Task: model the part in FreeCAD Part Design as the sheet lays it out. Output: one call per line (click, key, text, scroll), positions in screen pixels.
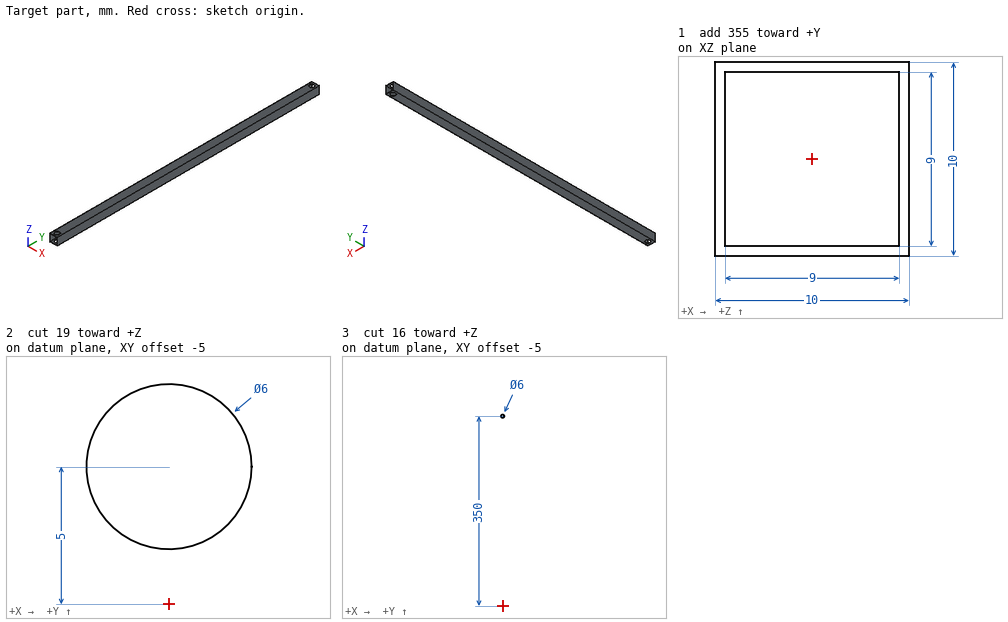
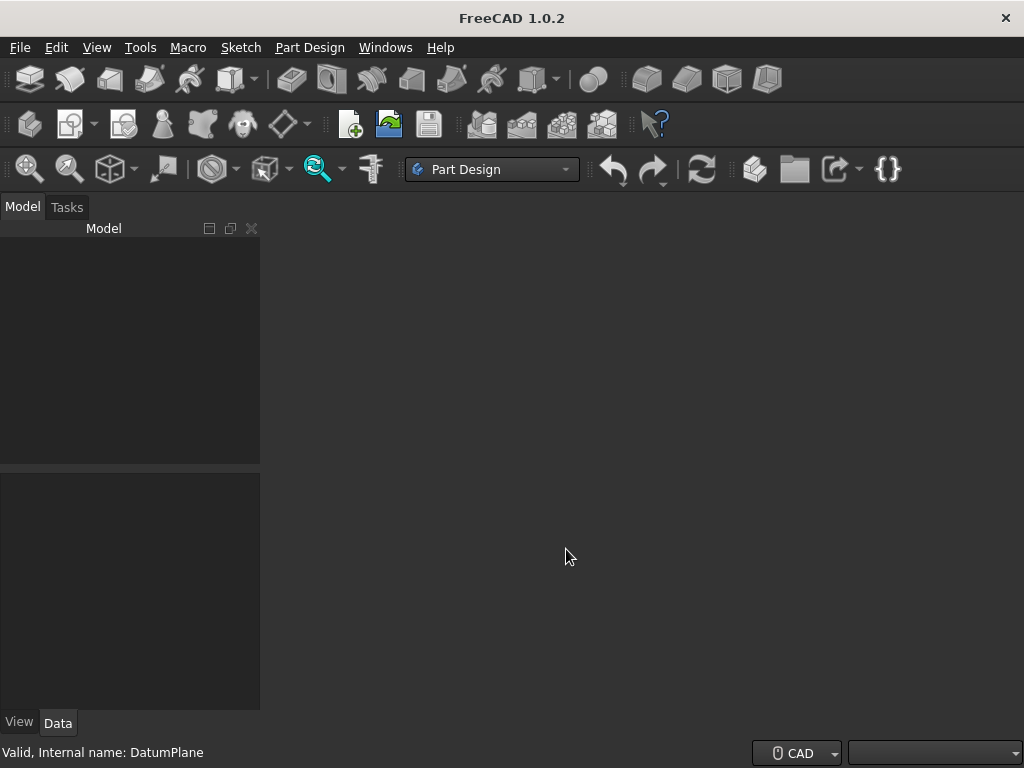
key(ctrl+n)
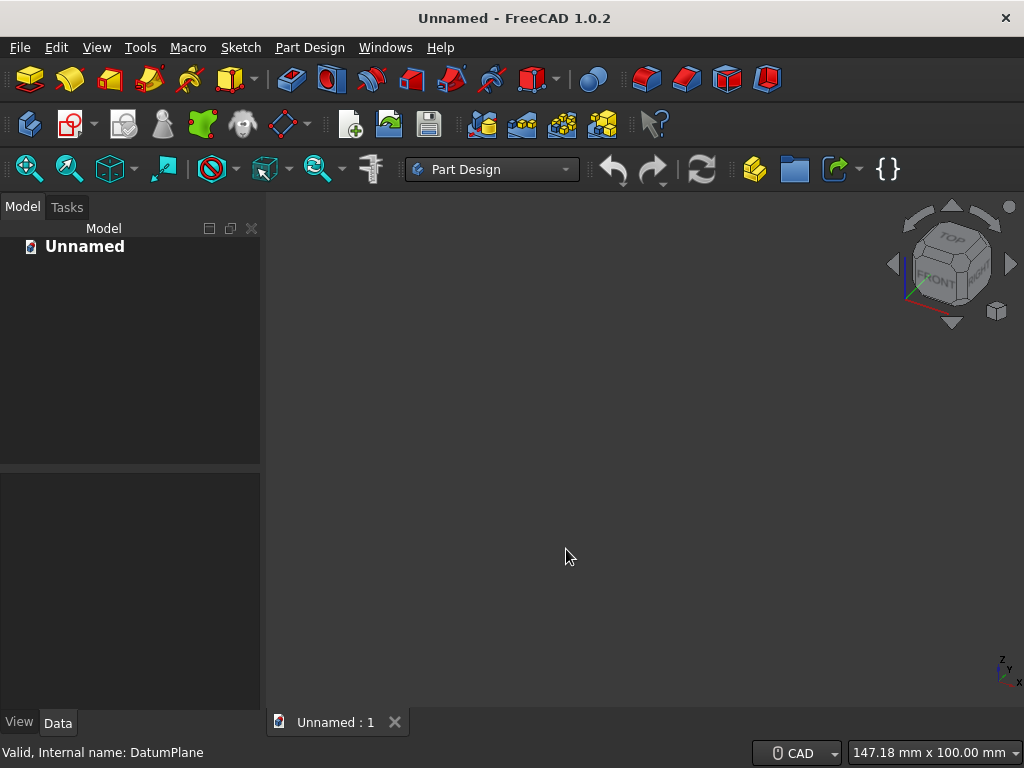
click(70, 124)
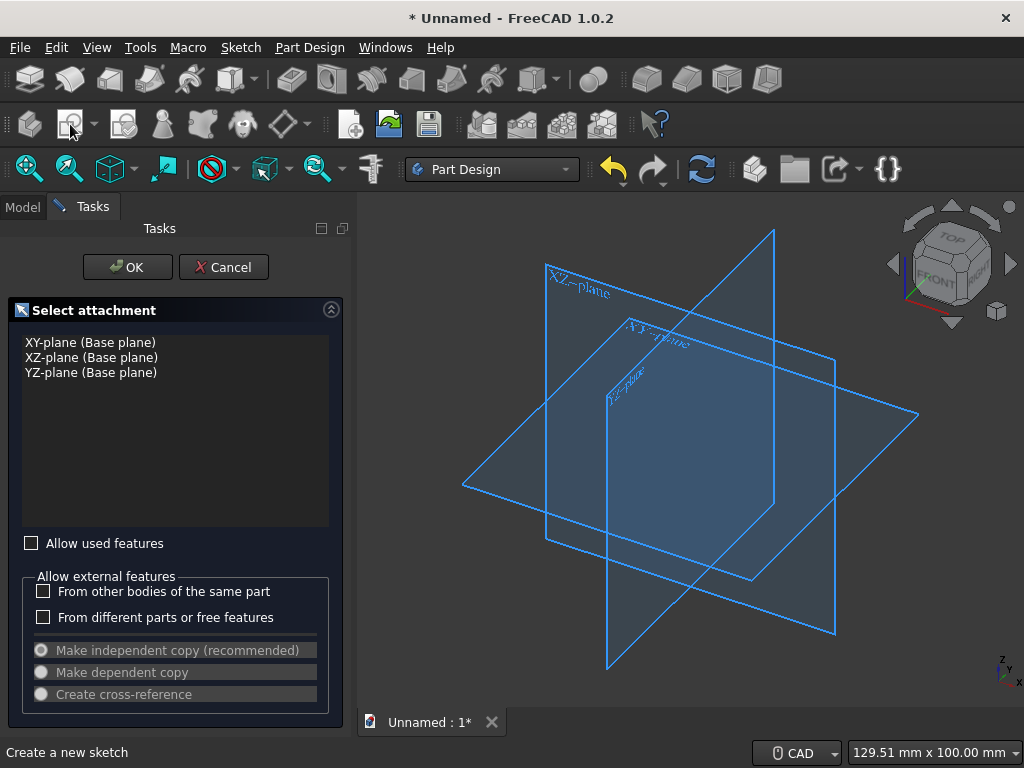
click(82, 358)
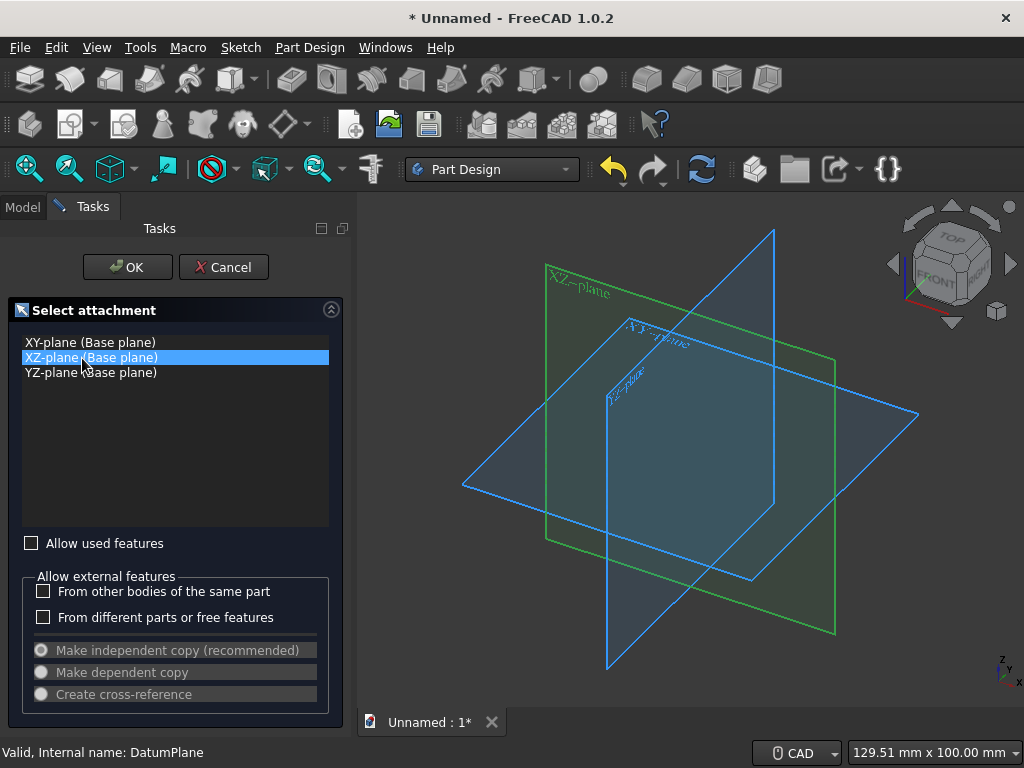
click(128, 267)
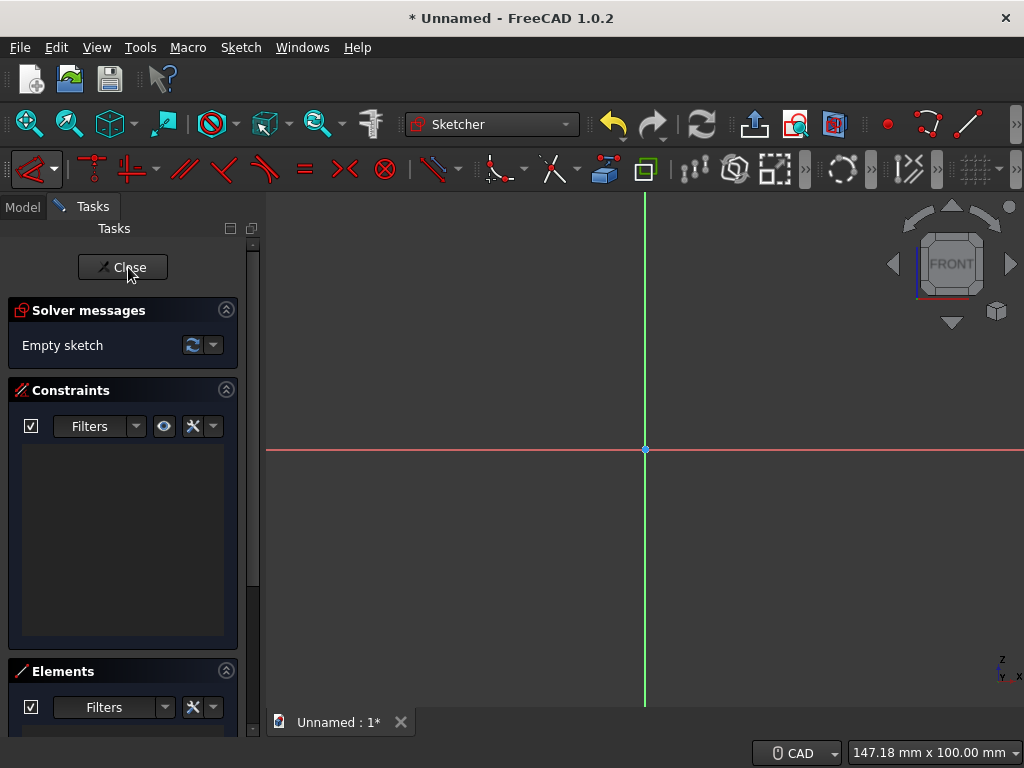
scroll(659, 450, up, 9)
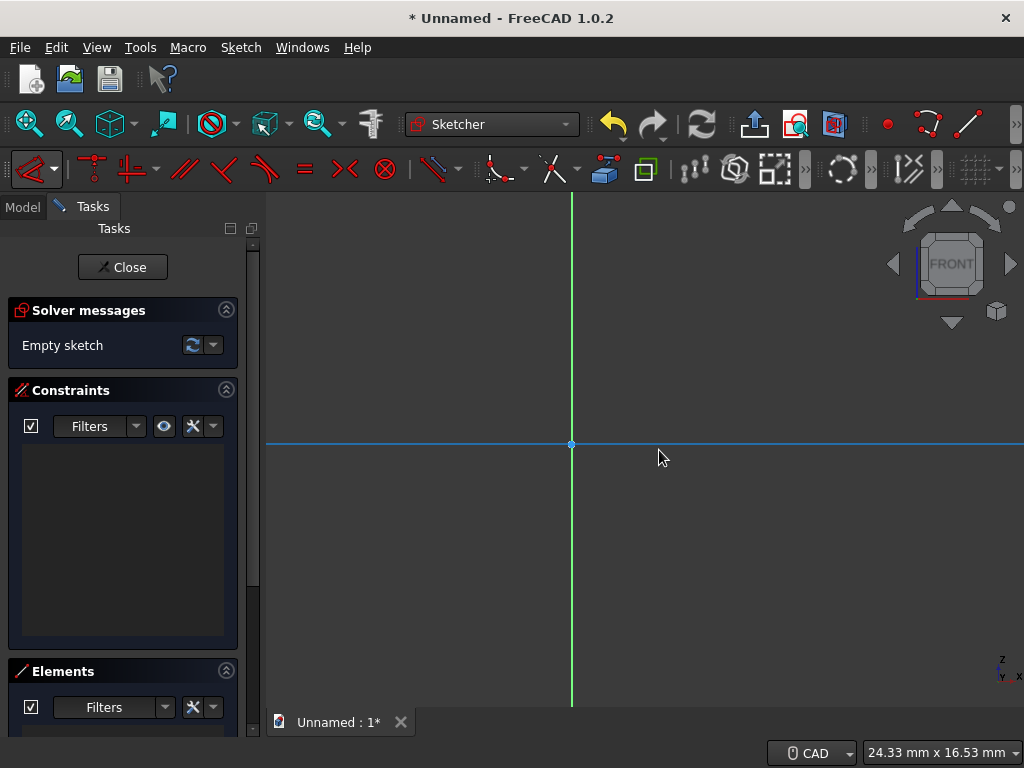
key(g)
key(v)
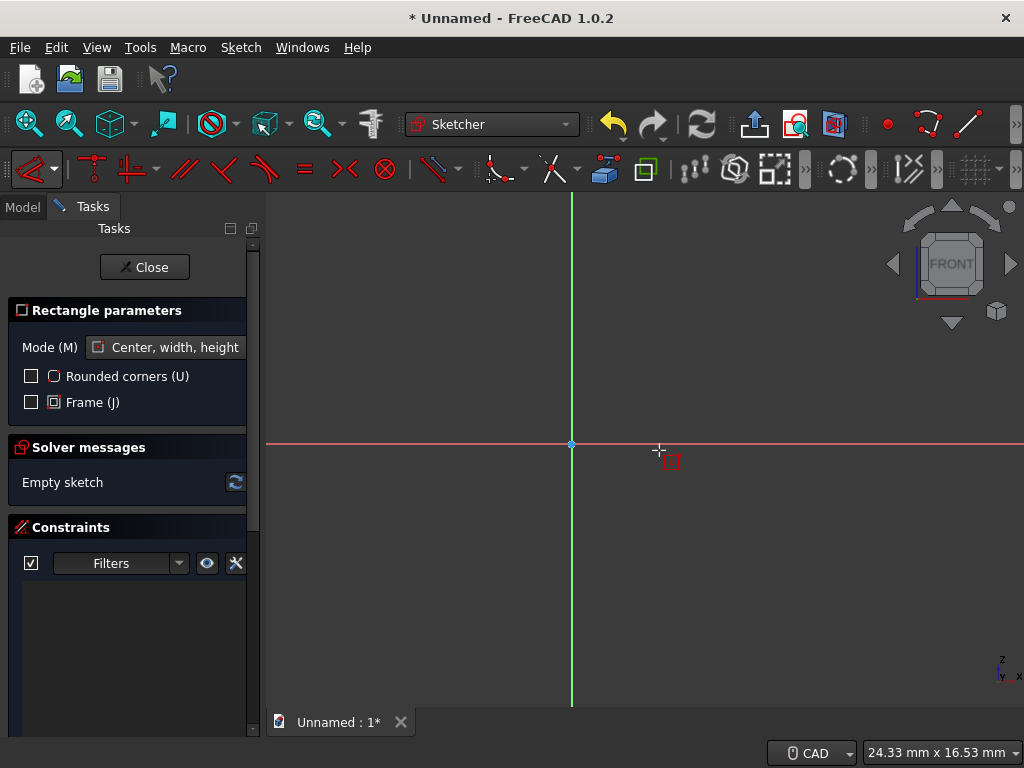
click(572, 444)
move(727, 289)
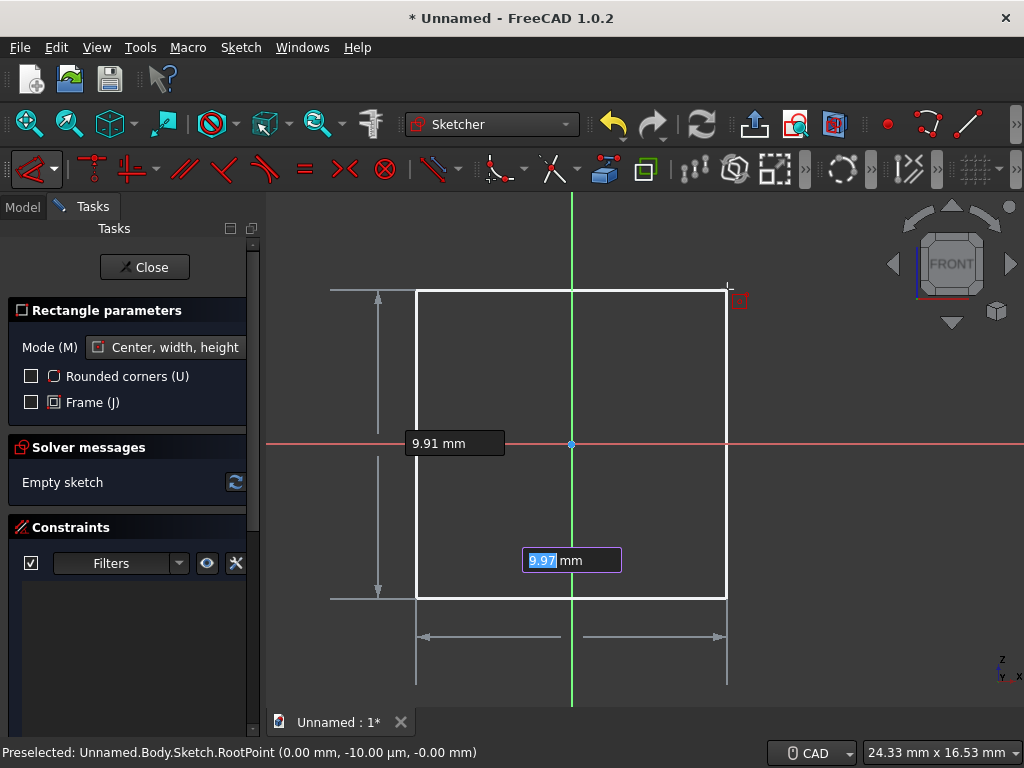
text(10)
key(Tab)
text(10)
key(Return)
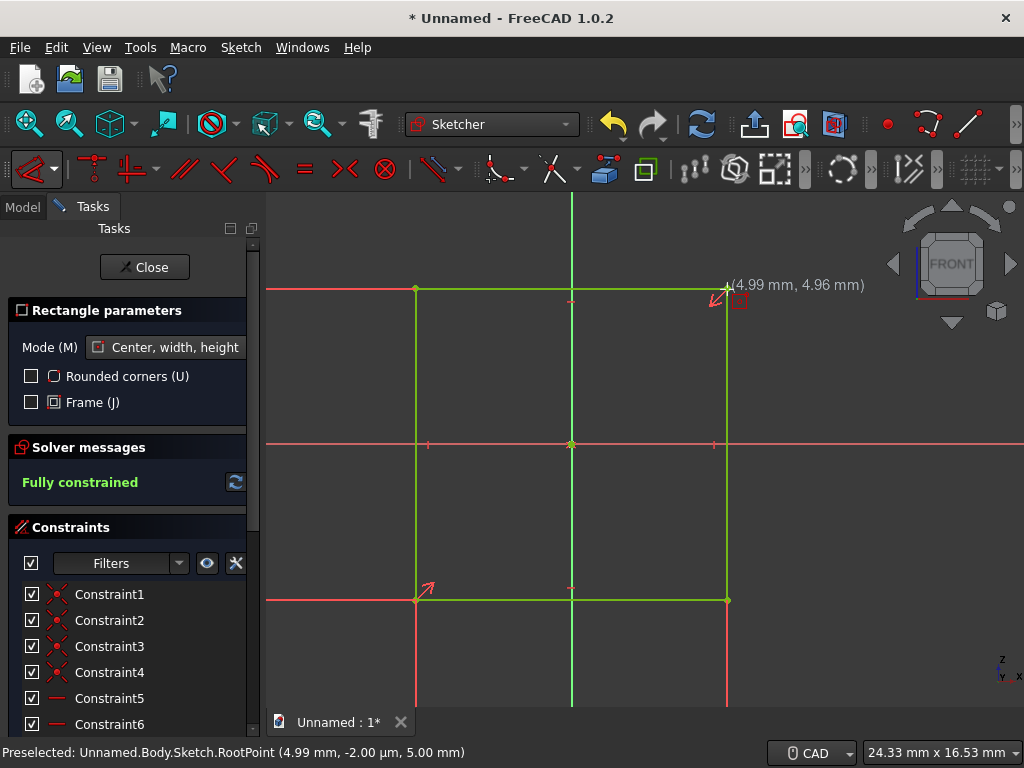
click(572, 444)
move(712, 304)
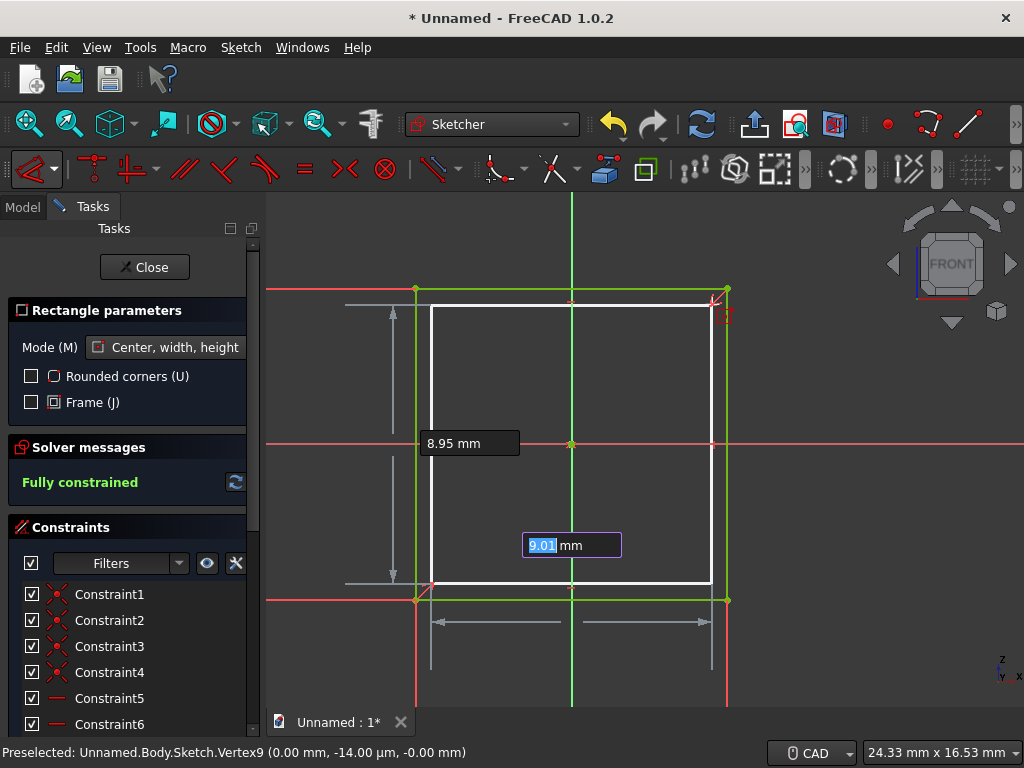
text(9)
key(Tab)
text(9)
key(Return)
key(Escape)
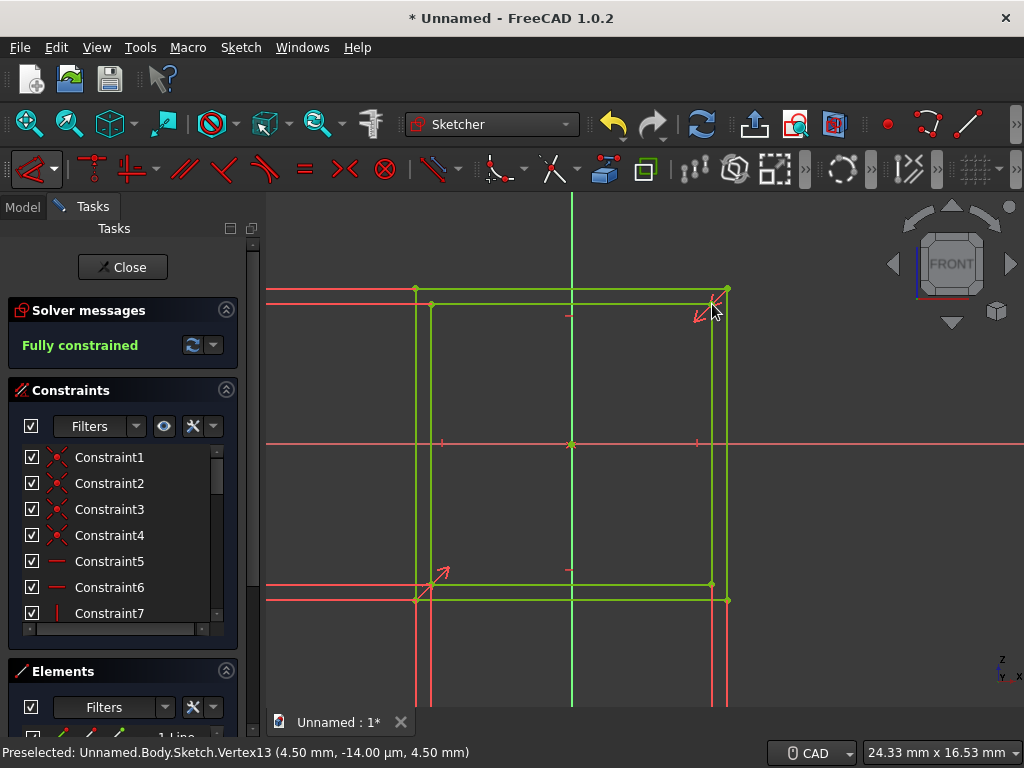
click(123, 267)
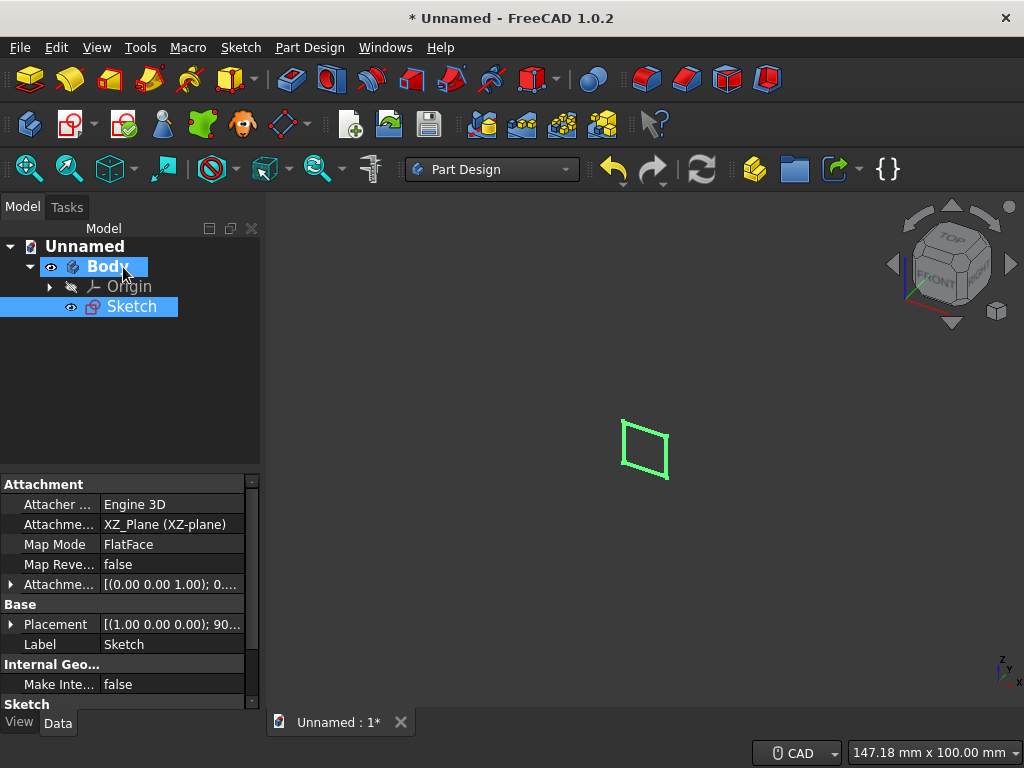
click(30, 80)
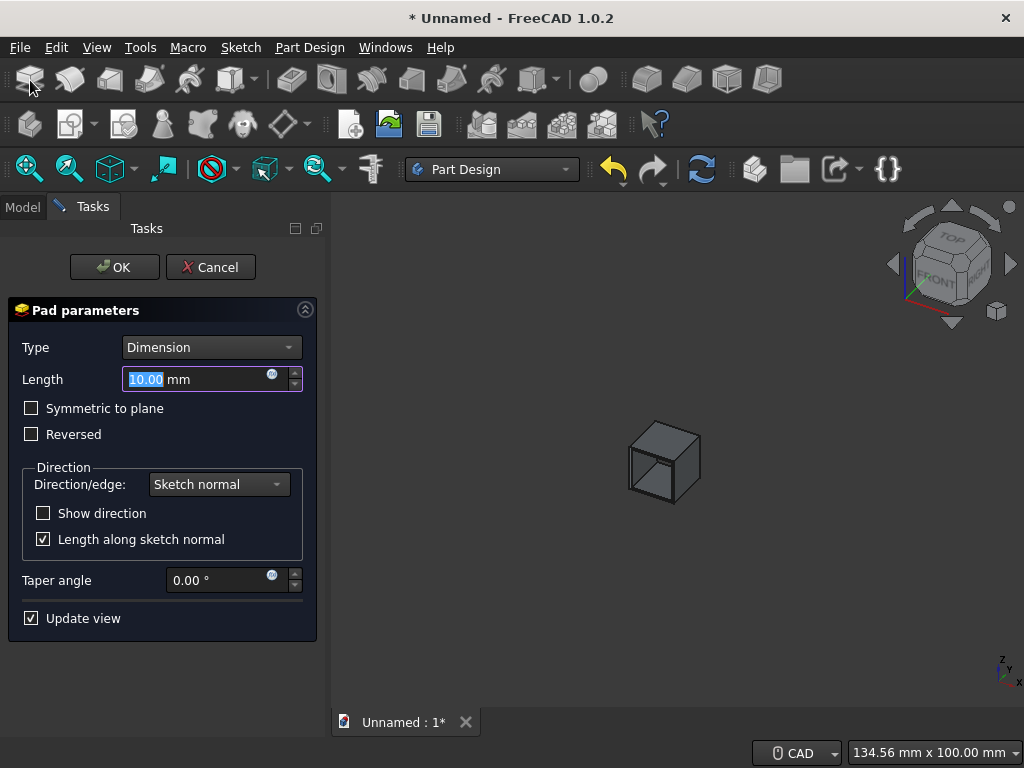
text(355)
key(Tab)